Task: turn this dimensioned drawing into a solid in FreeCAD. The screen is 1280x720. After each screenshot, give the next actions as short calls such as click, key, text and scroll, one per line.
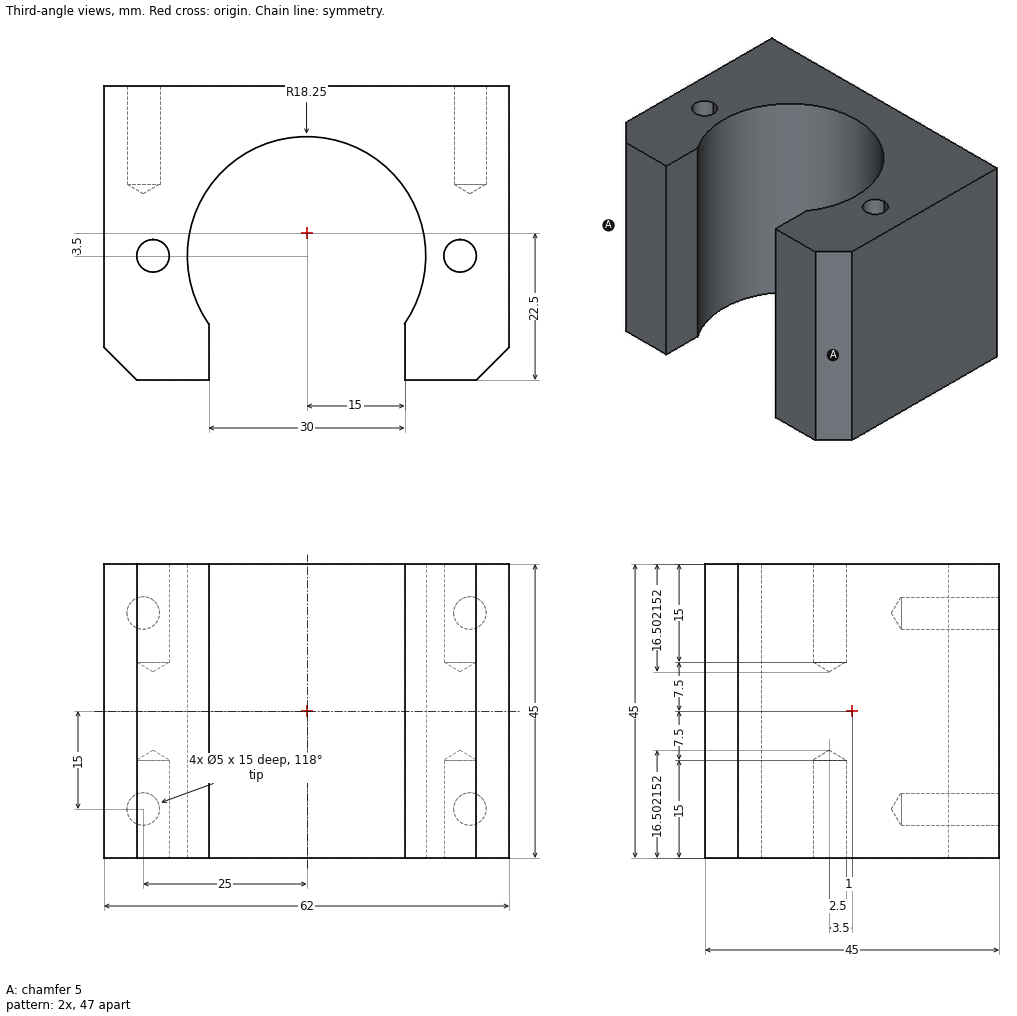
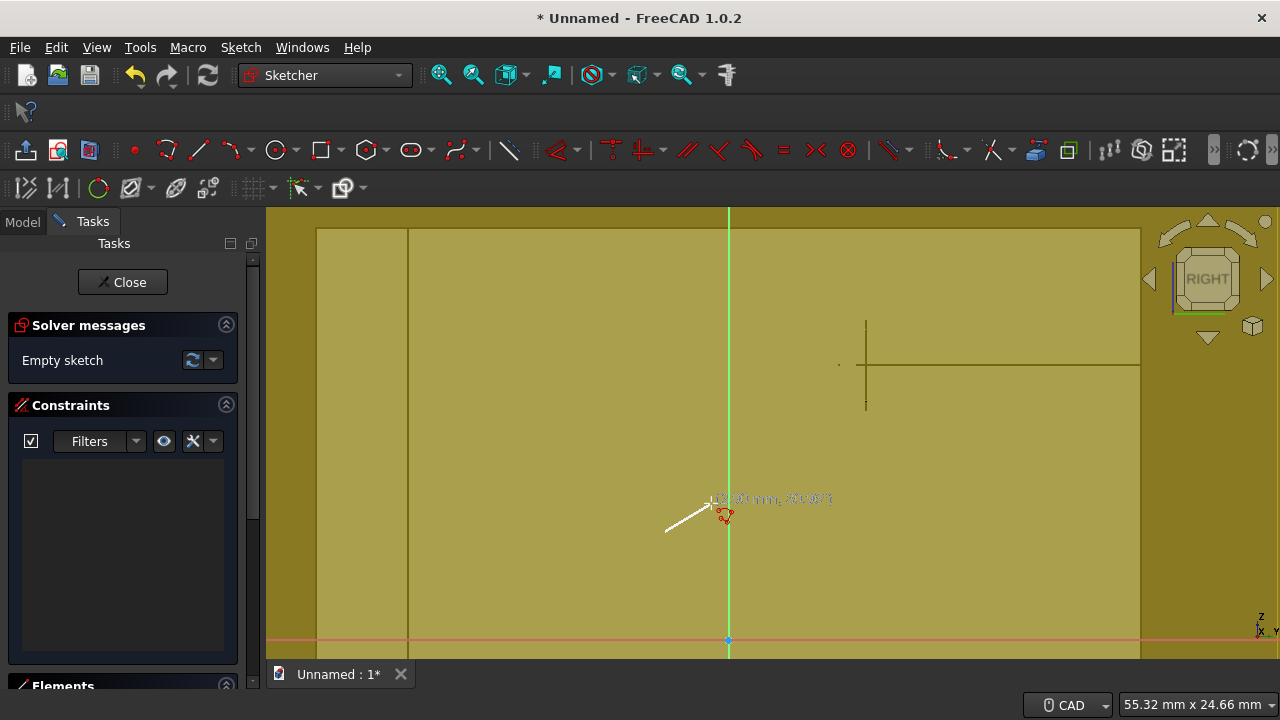
click(710, 503)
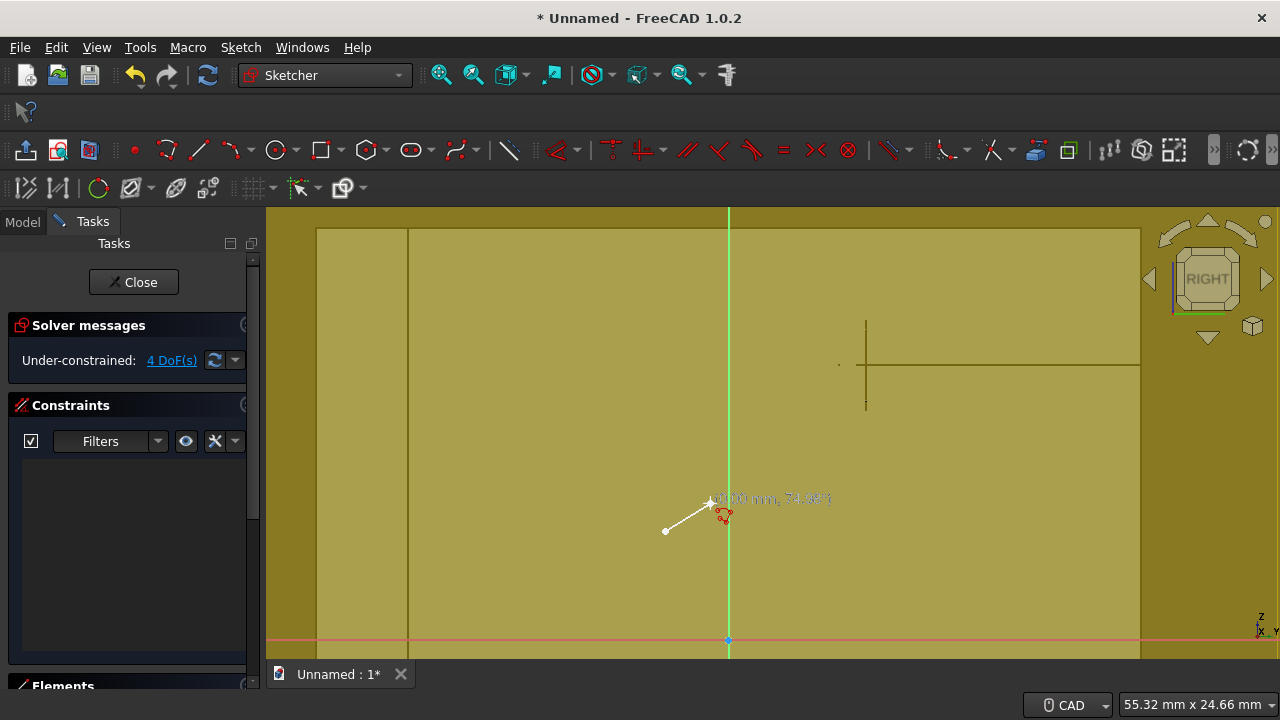
scroll(714, 505, down, 3)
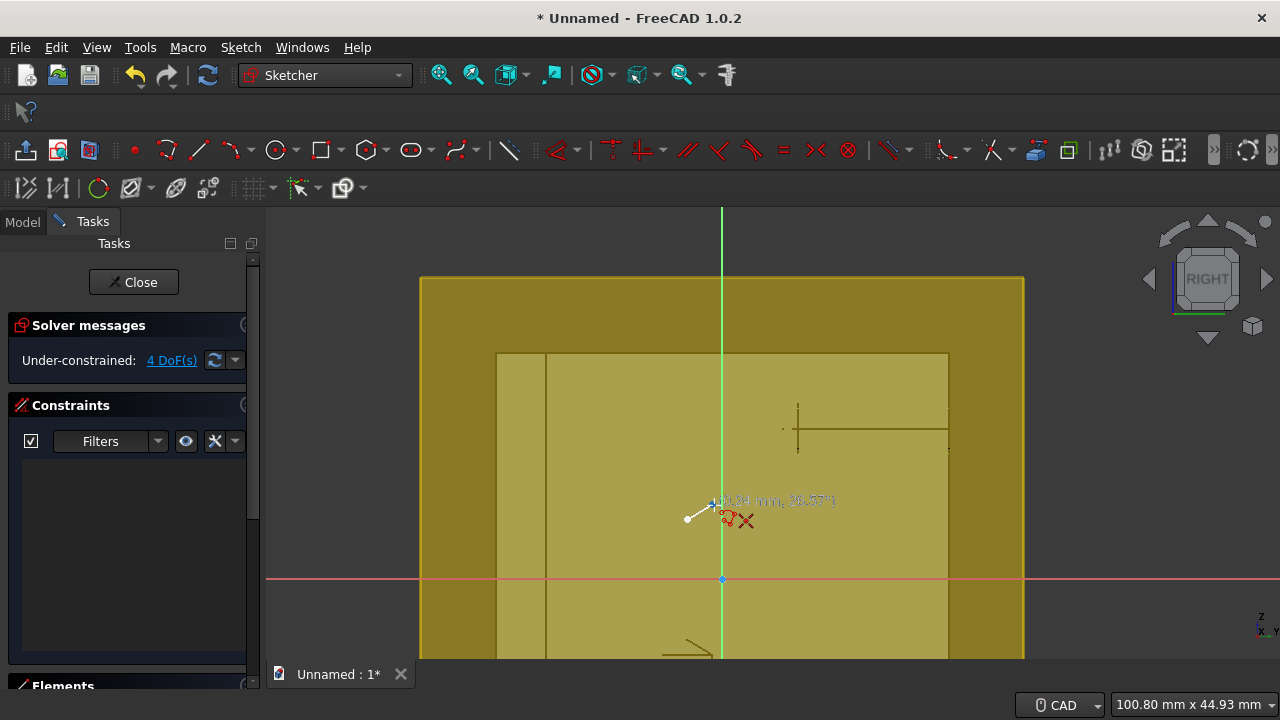
scroll(712, 353, up, 3)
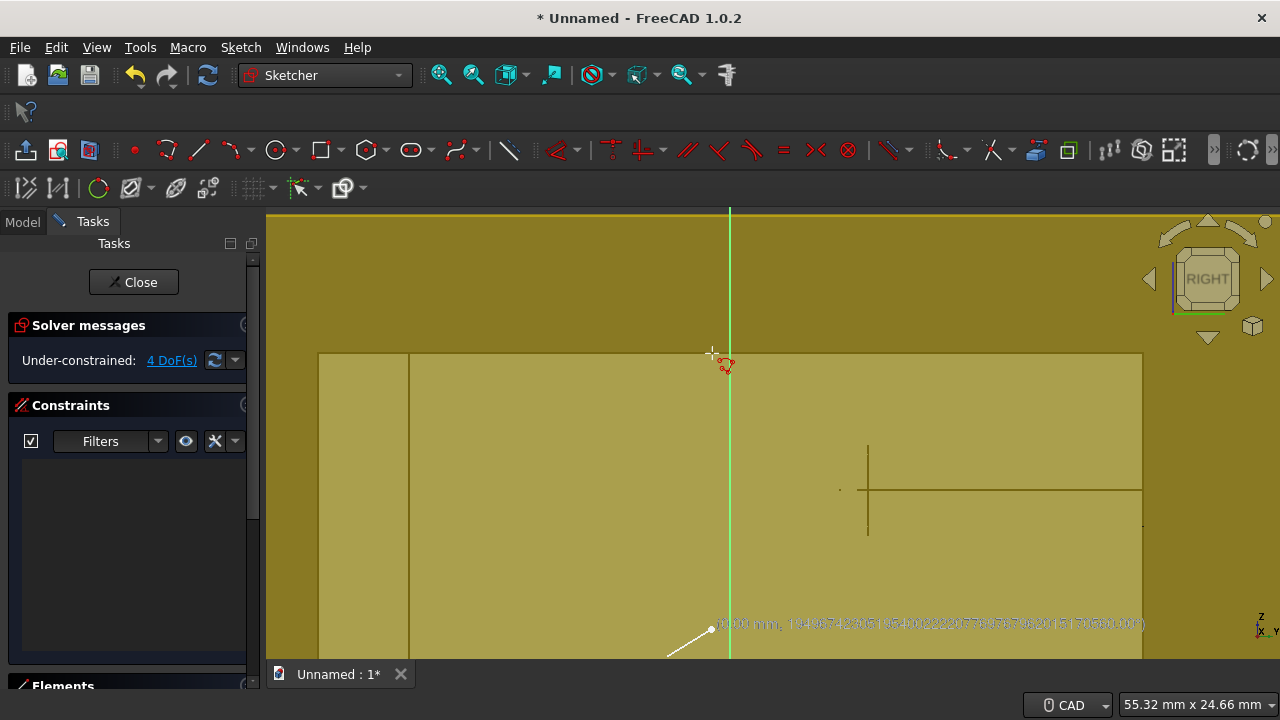
click(712, 353)
click(666, 353)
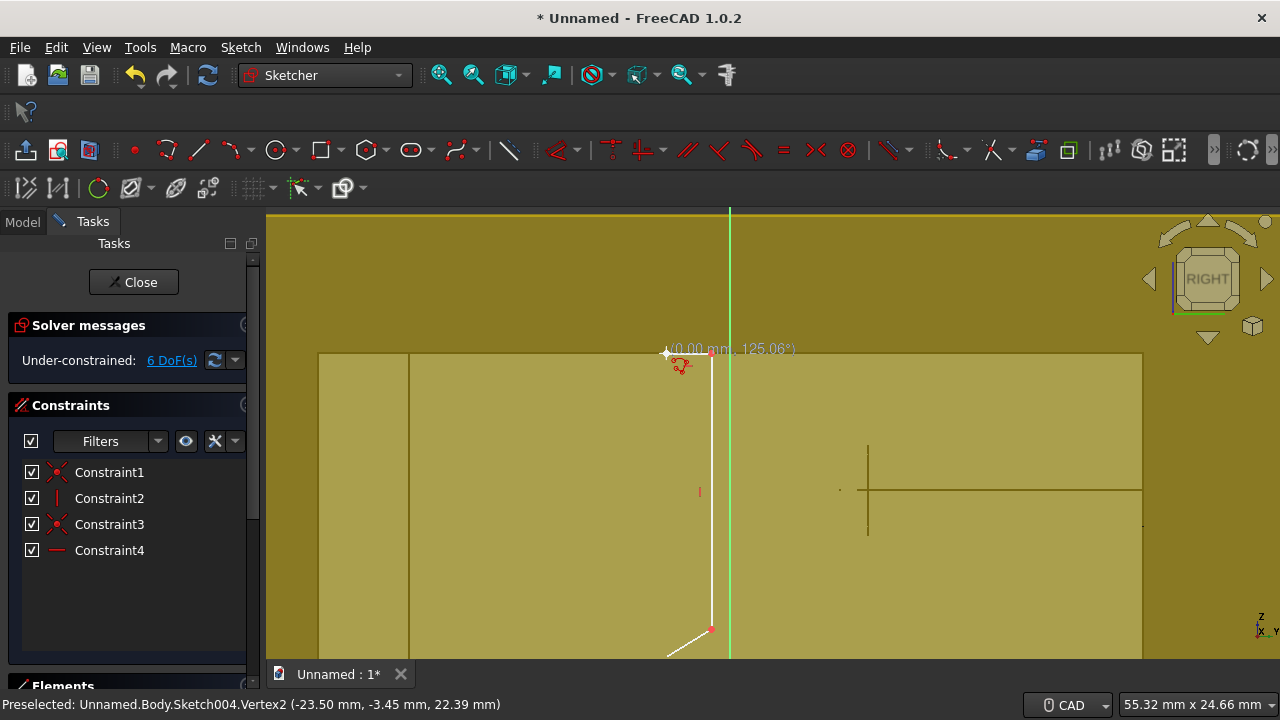
scroll(712, 353, down, 3)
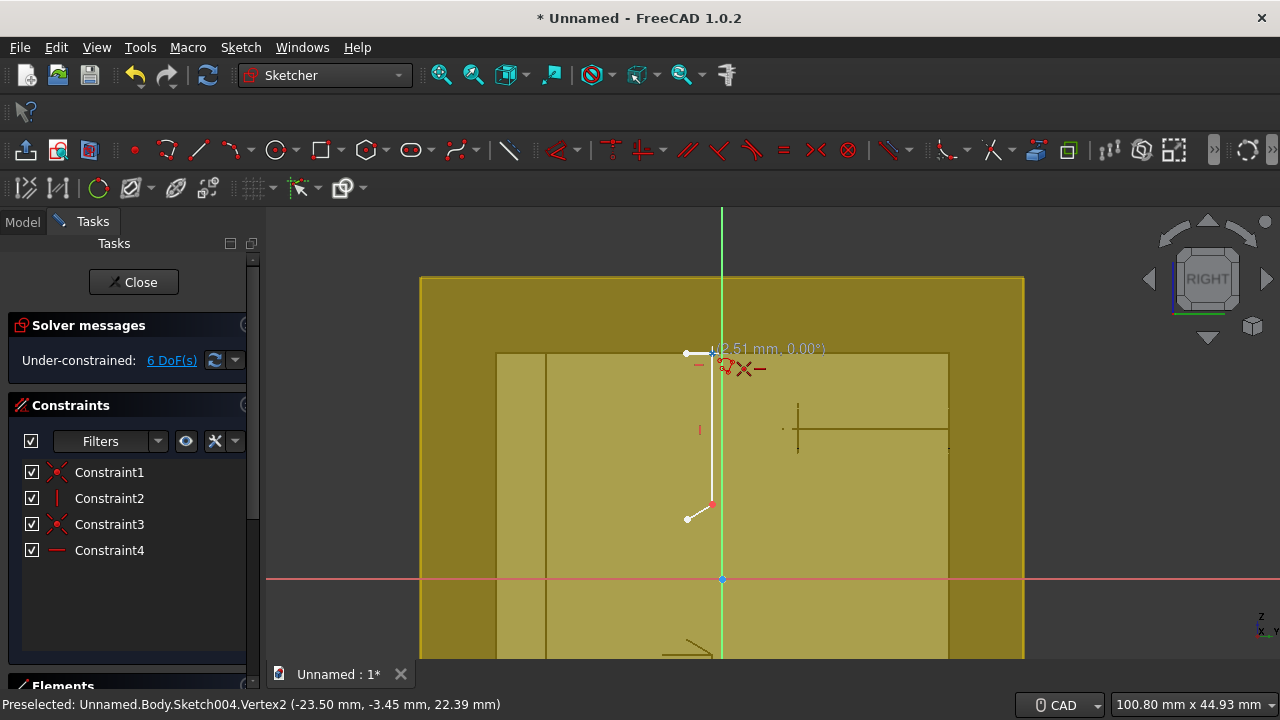
click(687, 520)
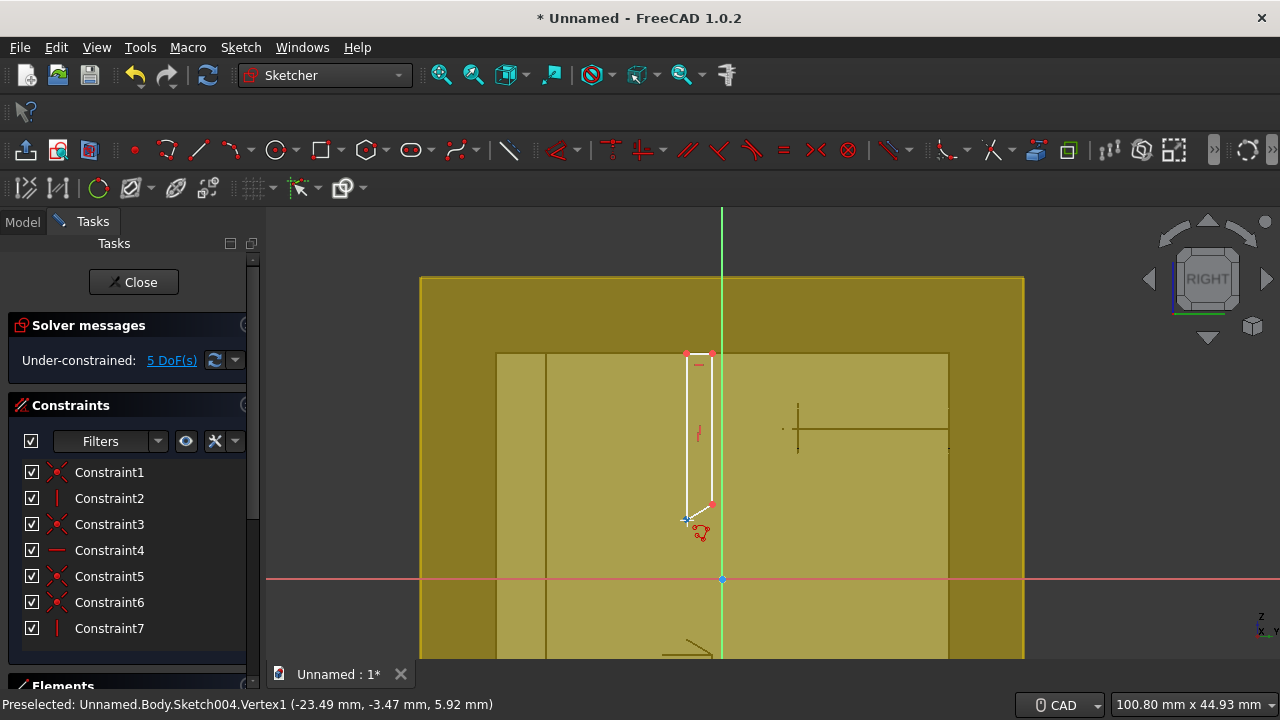
click(200, 150)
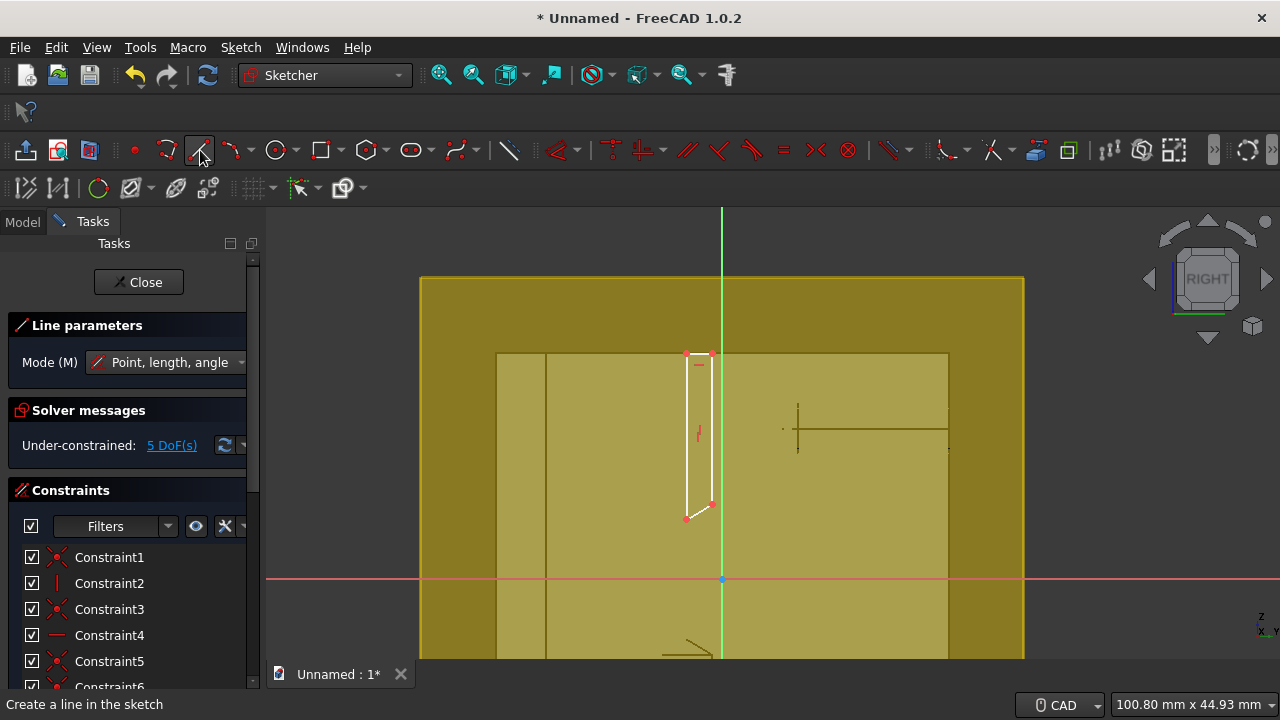
click(687, 337)
click(687, 287)
key(Escape)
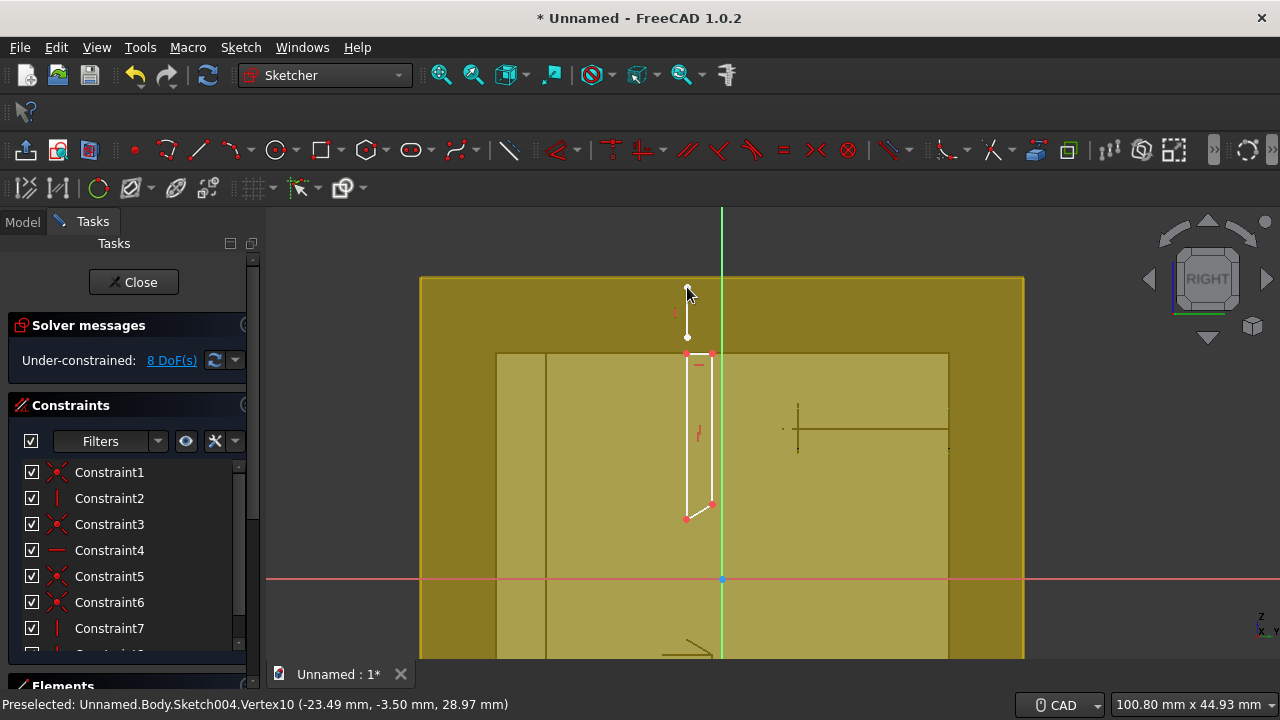
click(687, 323)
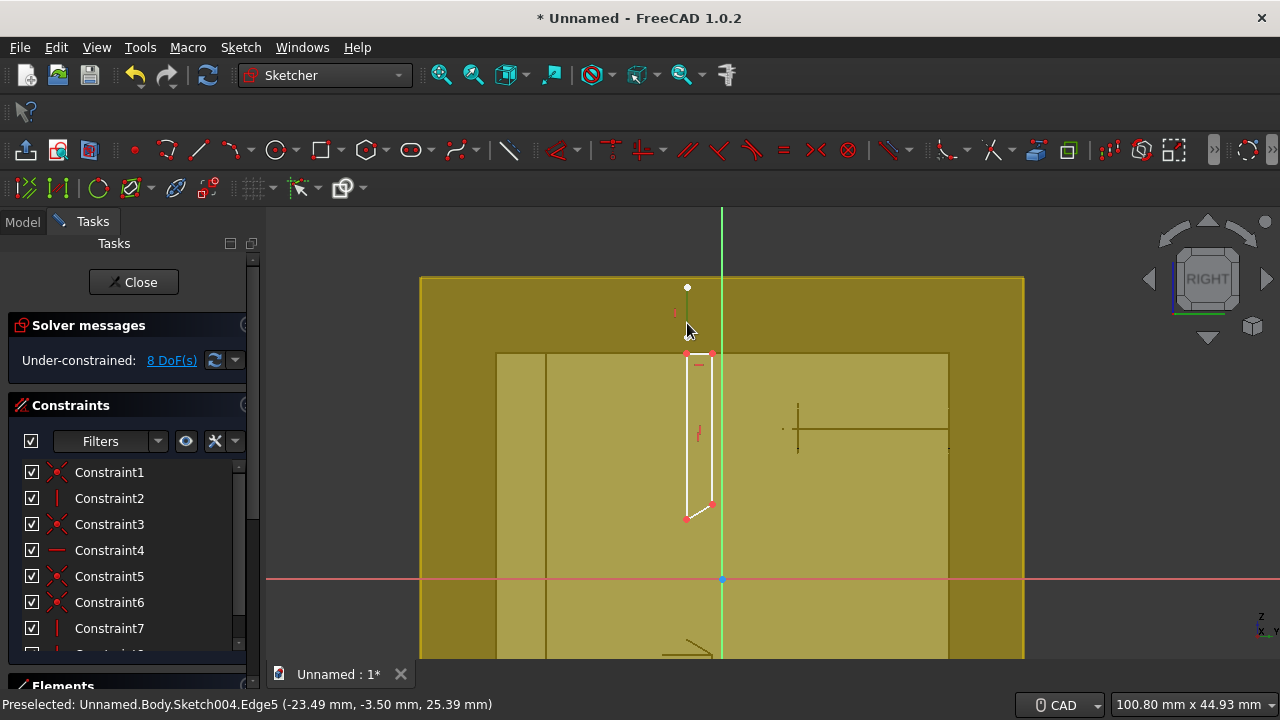
click(510, 150)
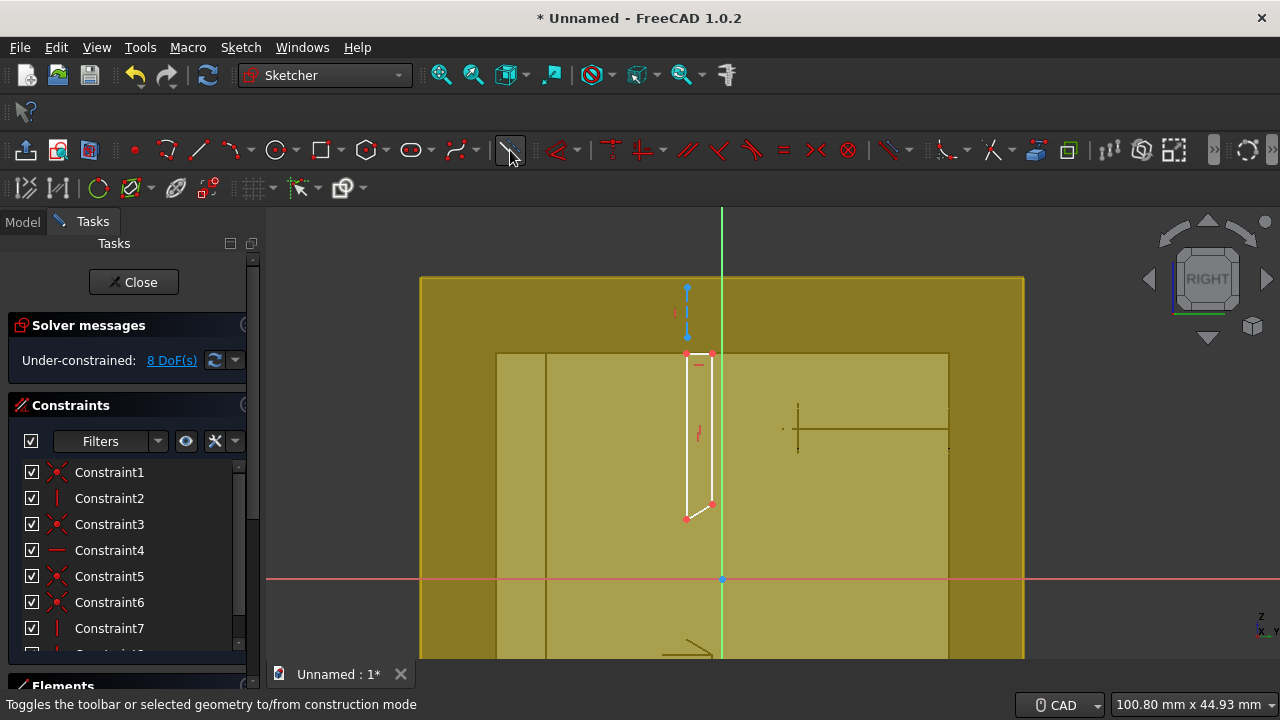
click(556, 150)